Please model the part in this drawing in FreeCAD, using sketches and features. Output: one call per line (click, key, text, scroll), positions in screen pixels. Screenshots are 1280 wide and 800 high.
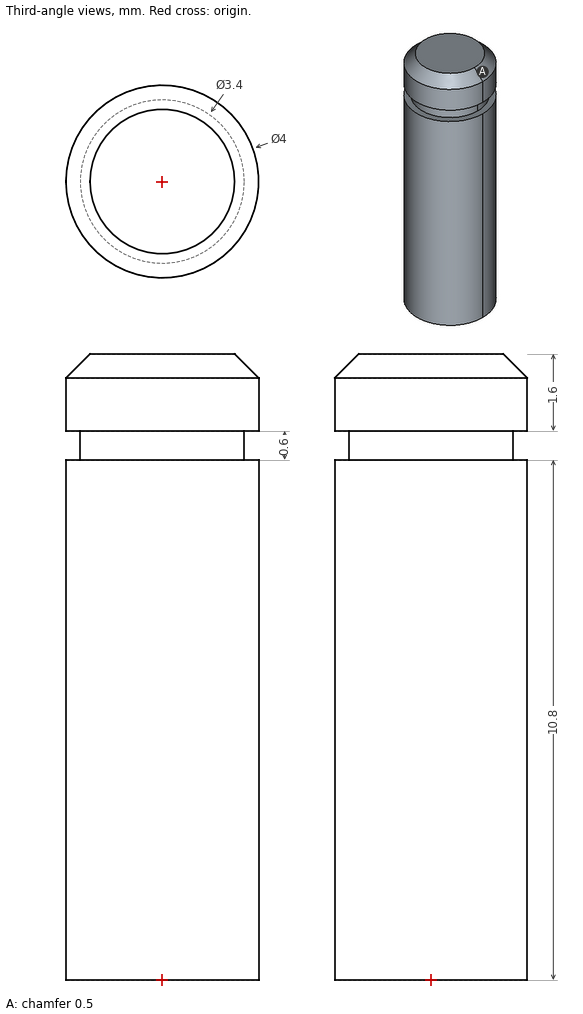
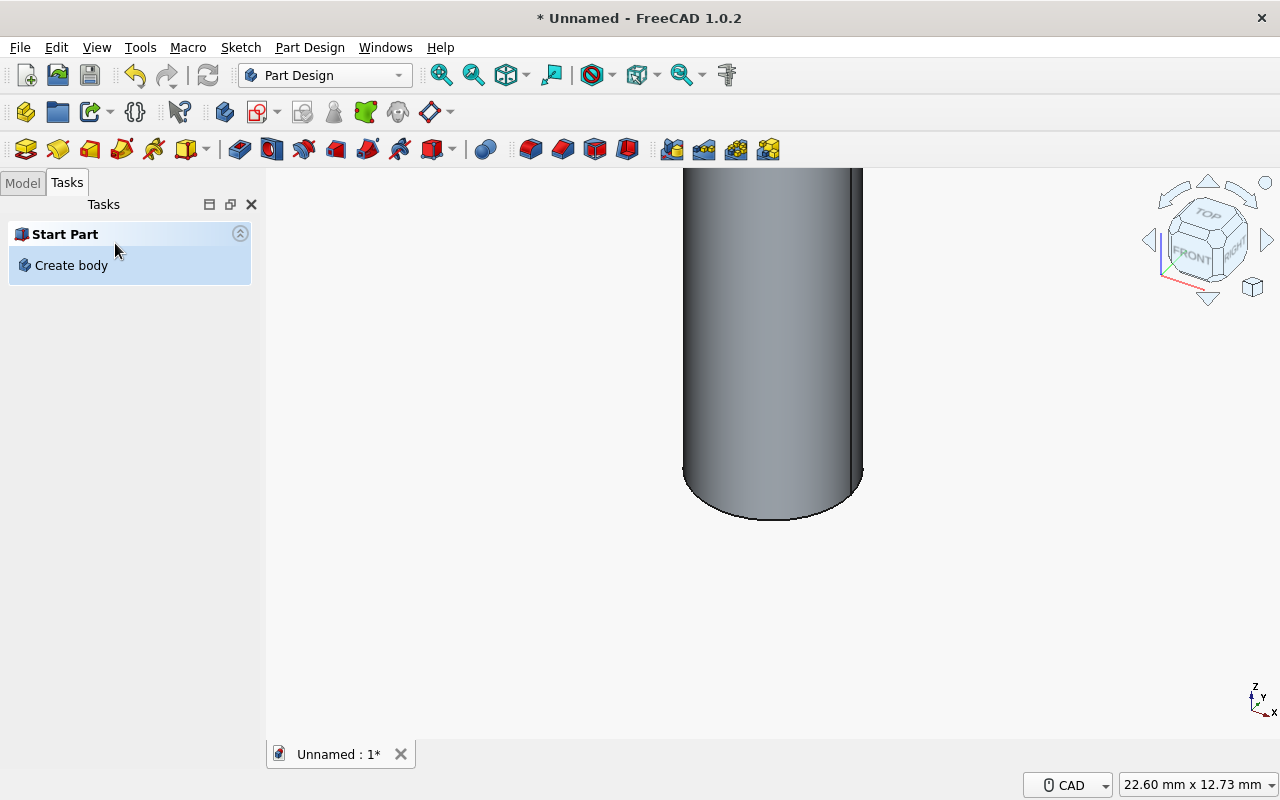
key(v)
key(f)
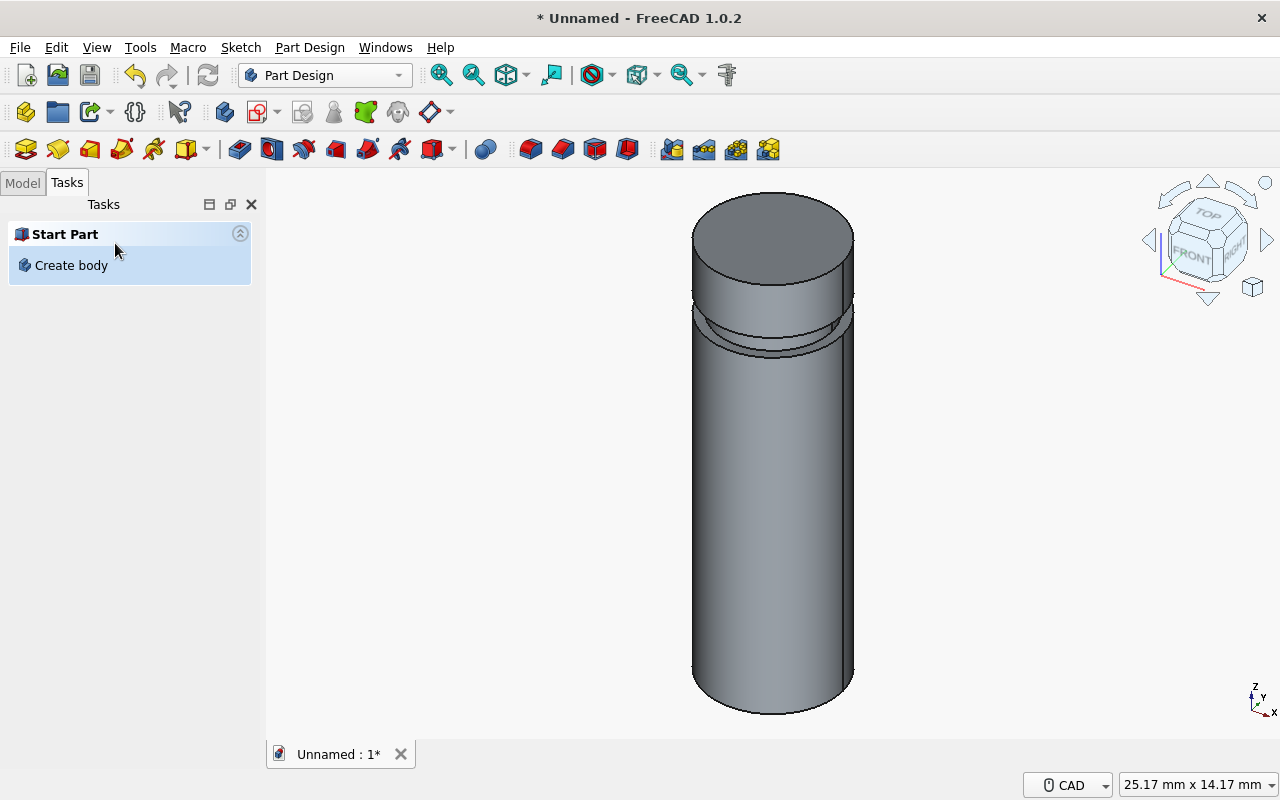
click(693, 243)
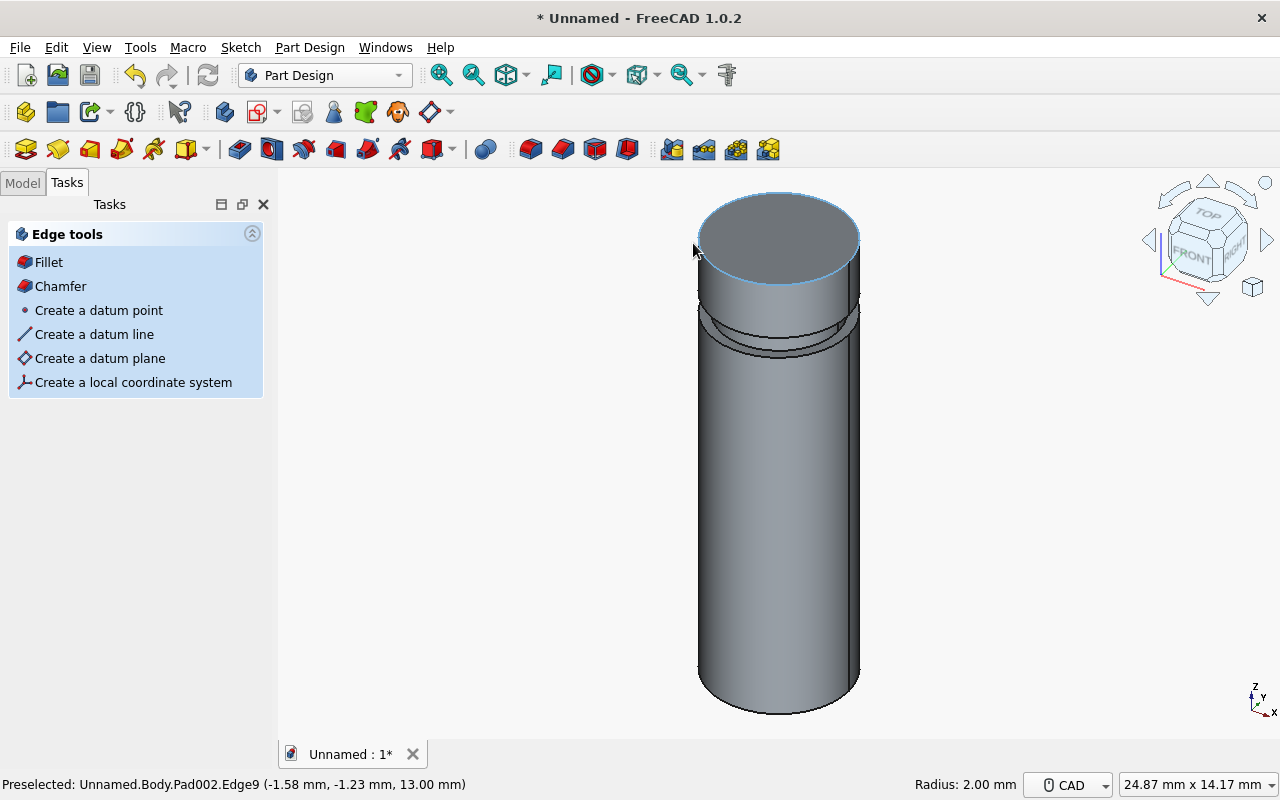
click(564, 150)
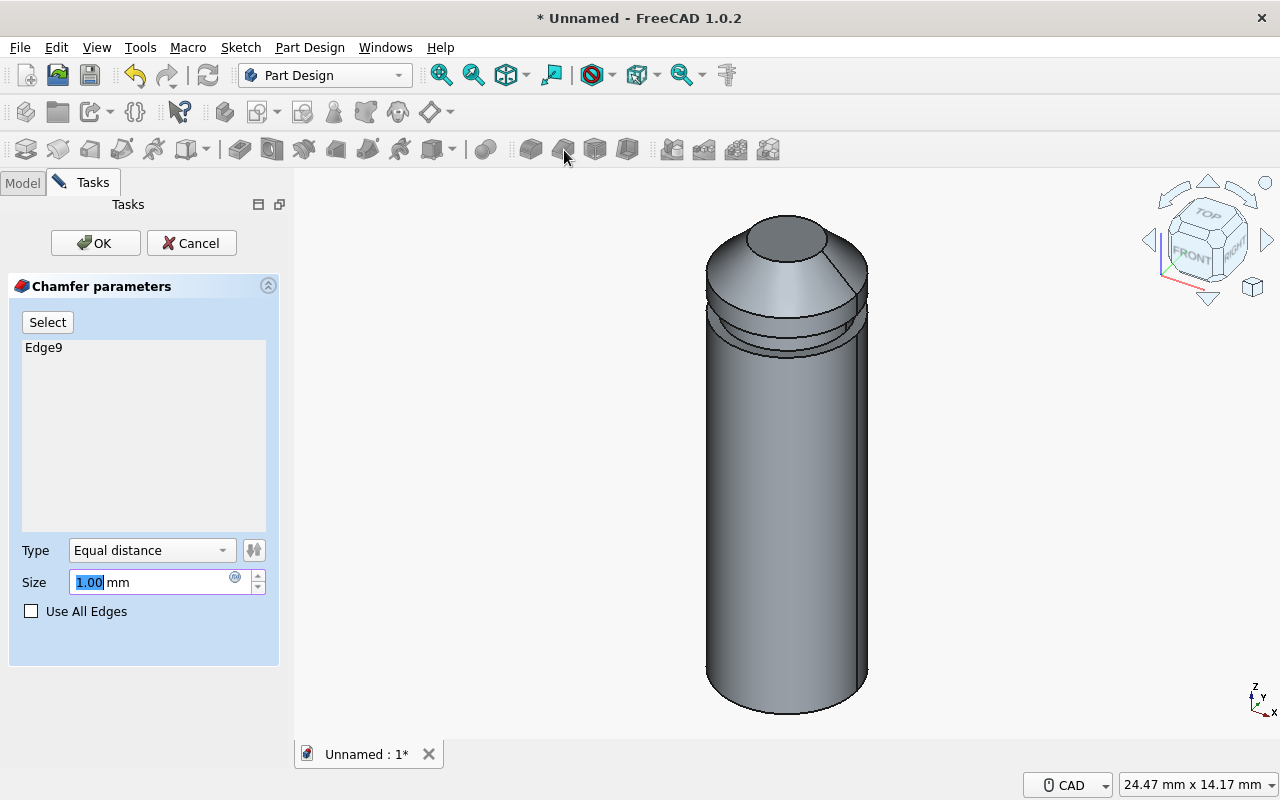
text(0.5)
key(Tab)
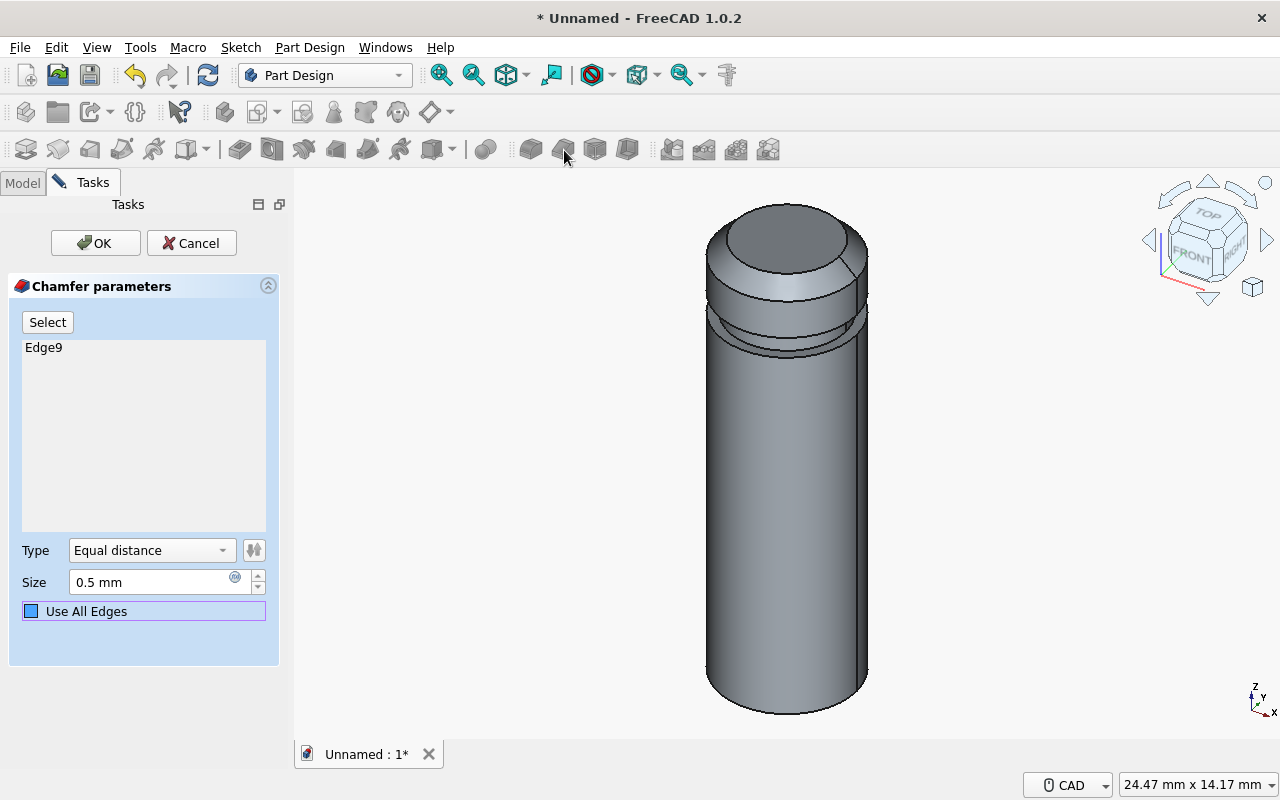
click(96, 243)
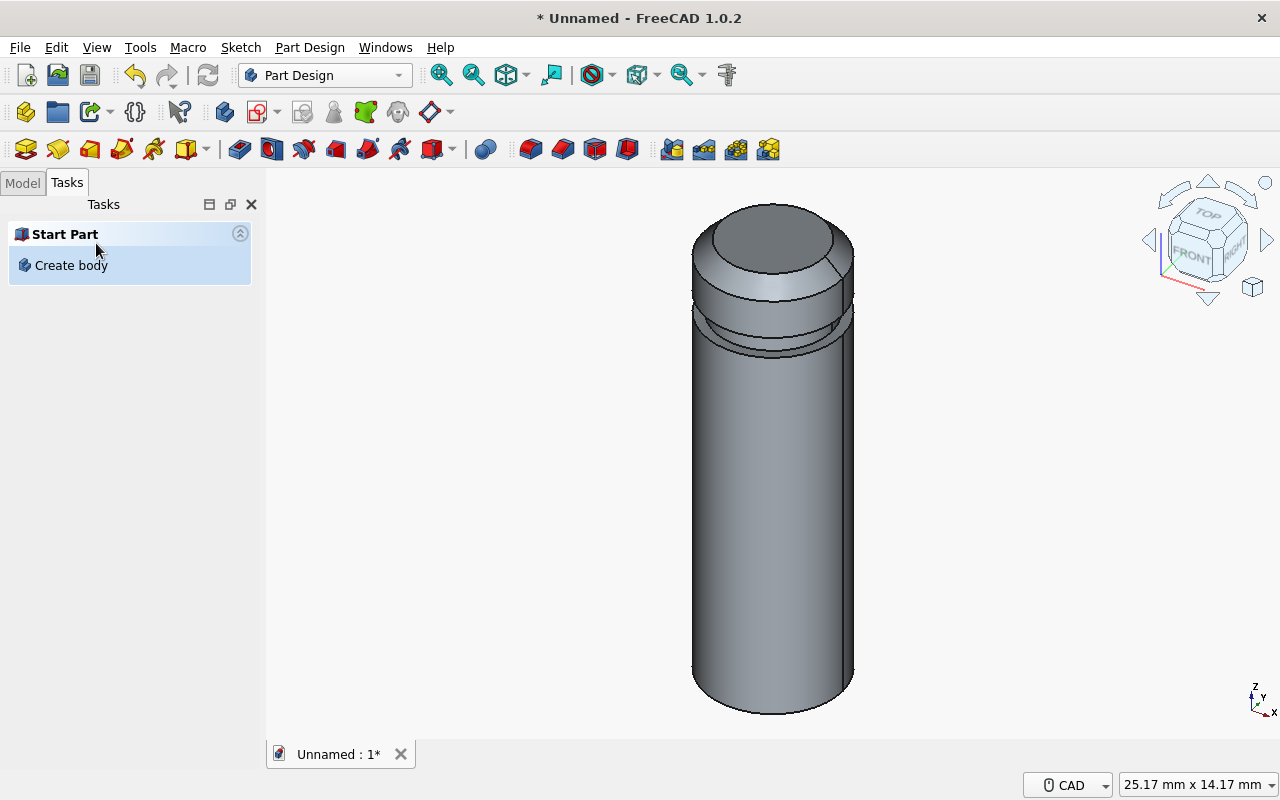
key(0)